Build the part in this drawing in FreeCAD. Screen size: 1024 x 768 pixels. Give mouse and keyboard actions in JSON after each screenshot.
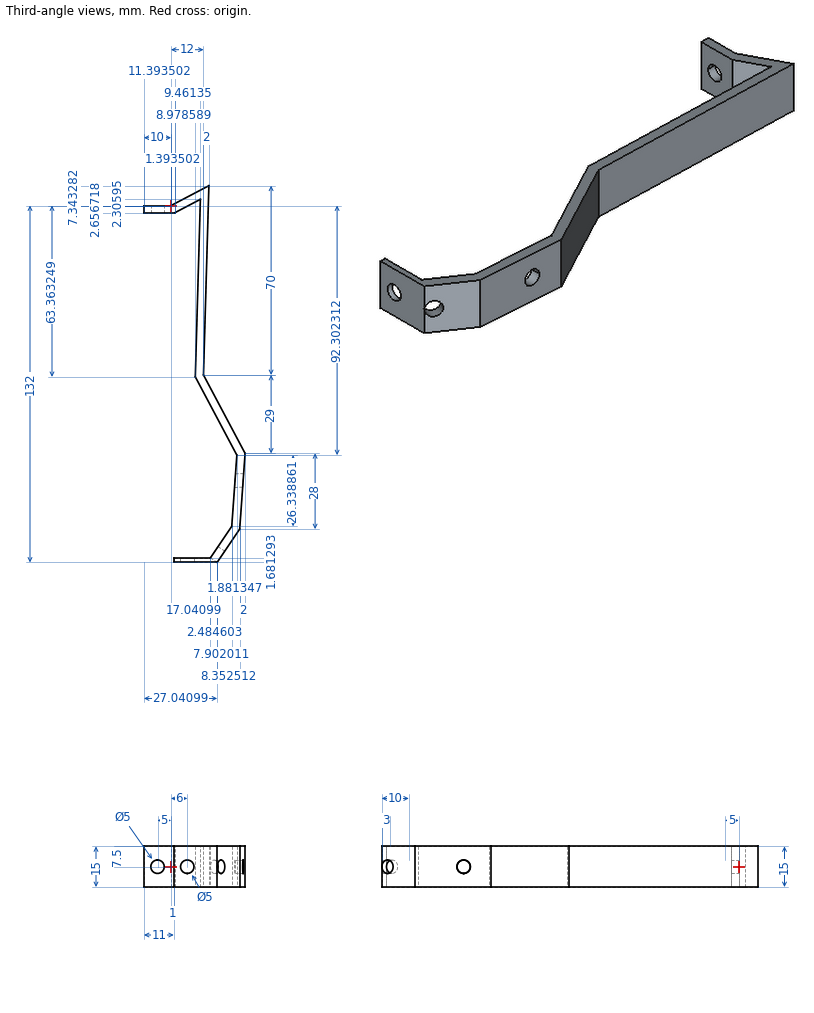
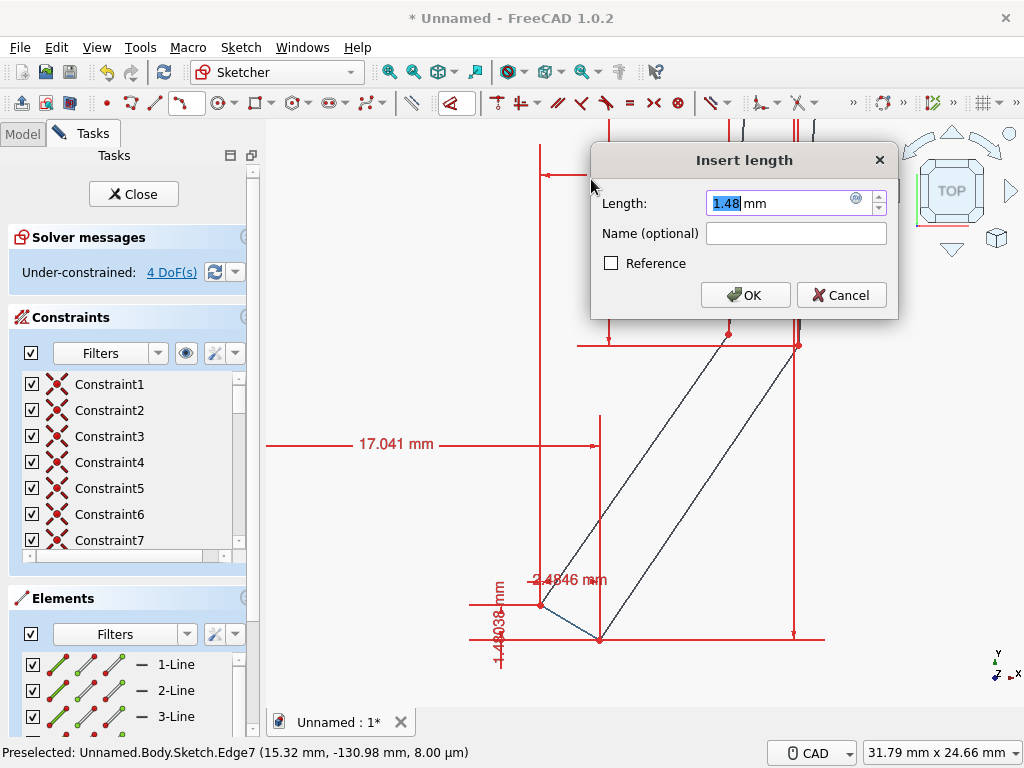
{"action": "type", "text": "1.681293"}
{"action": "key", "text": "Return"}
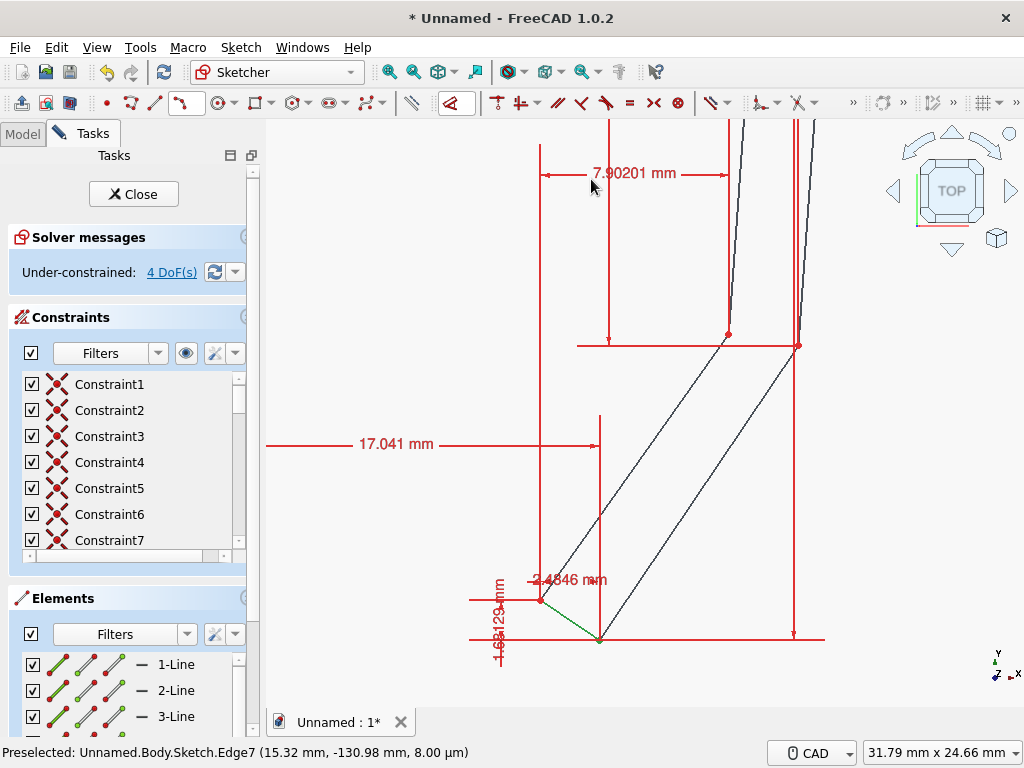
{"action": "scroll", "coordinate": [584, 592], "scroll_direction": "down", "scroll_amount": 11}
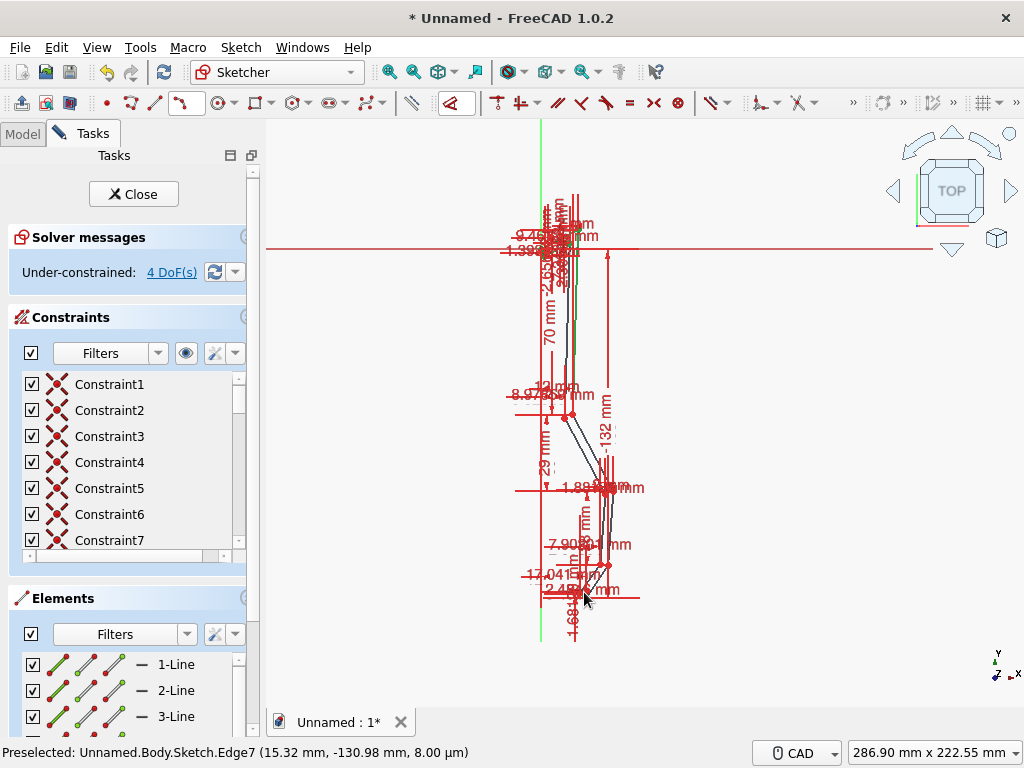
{"action": "scroll", "coordinate": [593, 588], "scroll_direction": "up", "scroll_amount": 3}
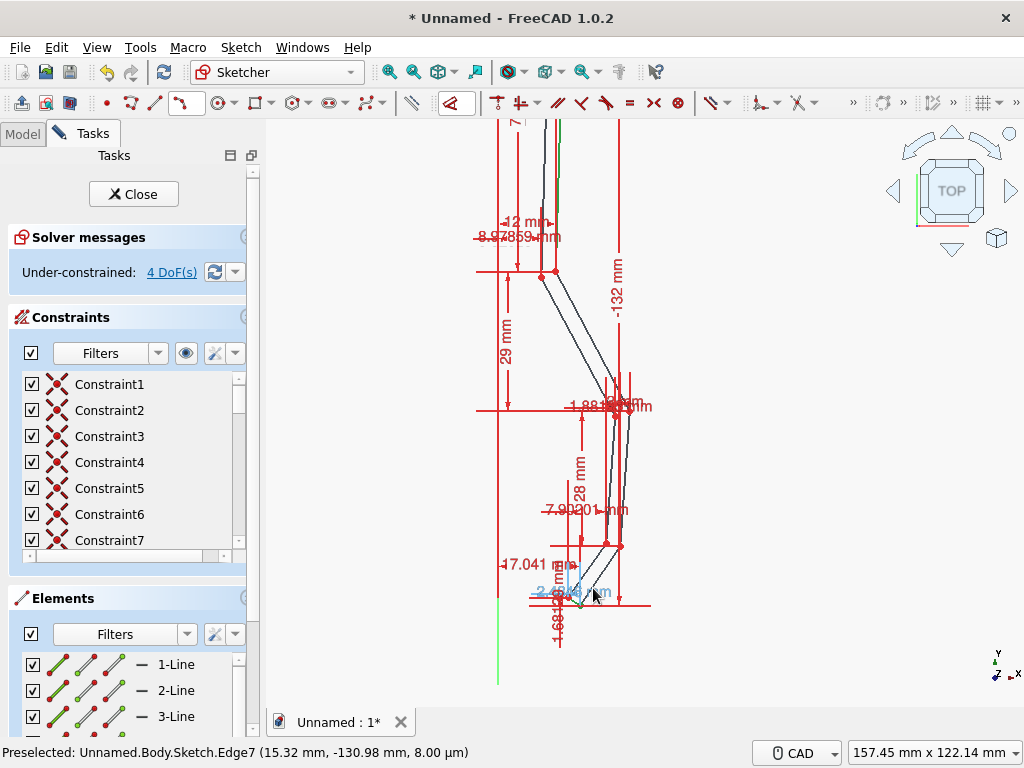
{"action": "left_click", "coordinate": [608, 564]}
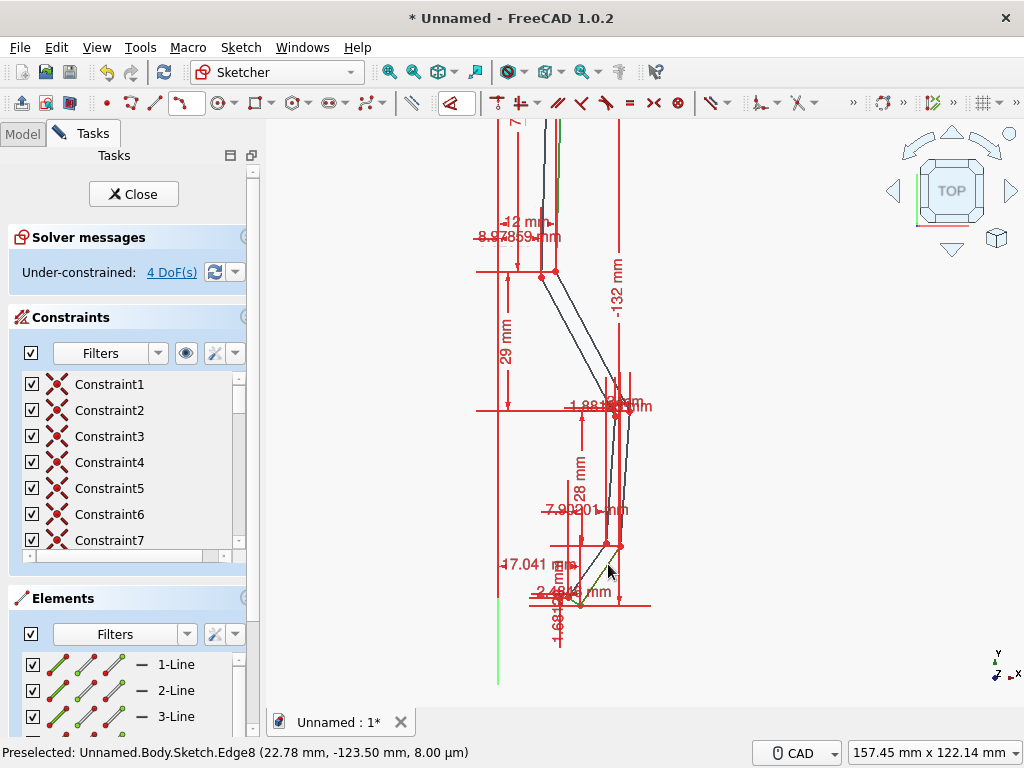
{"action": "left_click", "coordinate": [470, 104]}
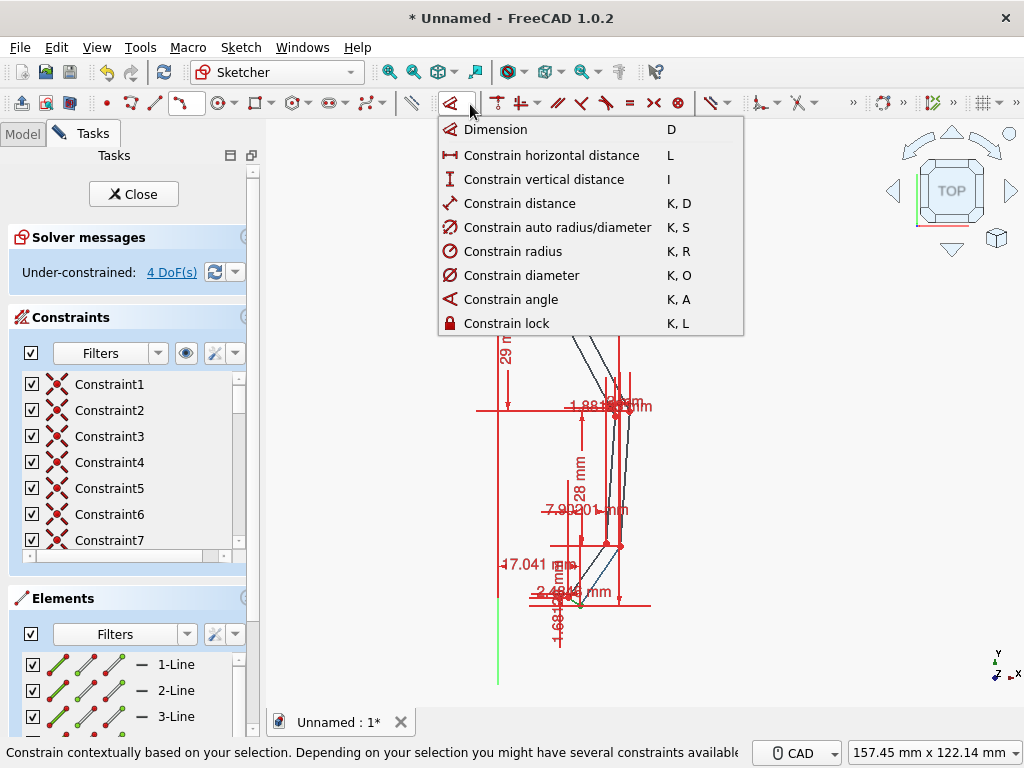
{"action": "left_click", "coordinate": [591, 155]}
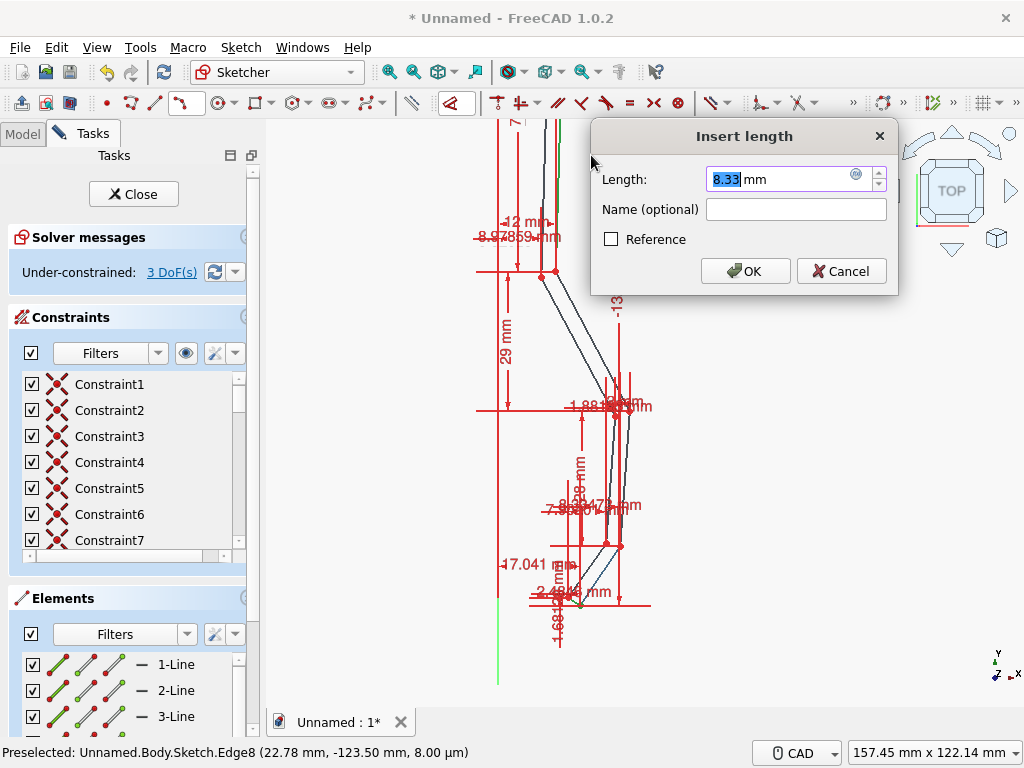
{"action": "type", "text": "8.352512"}
{"action": "key", "text": "Return"}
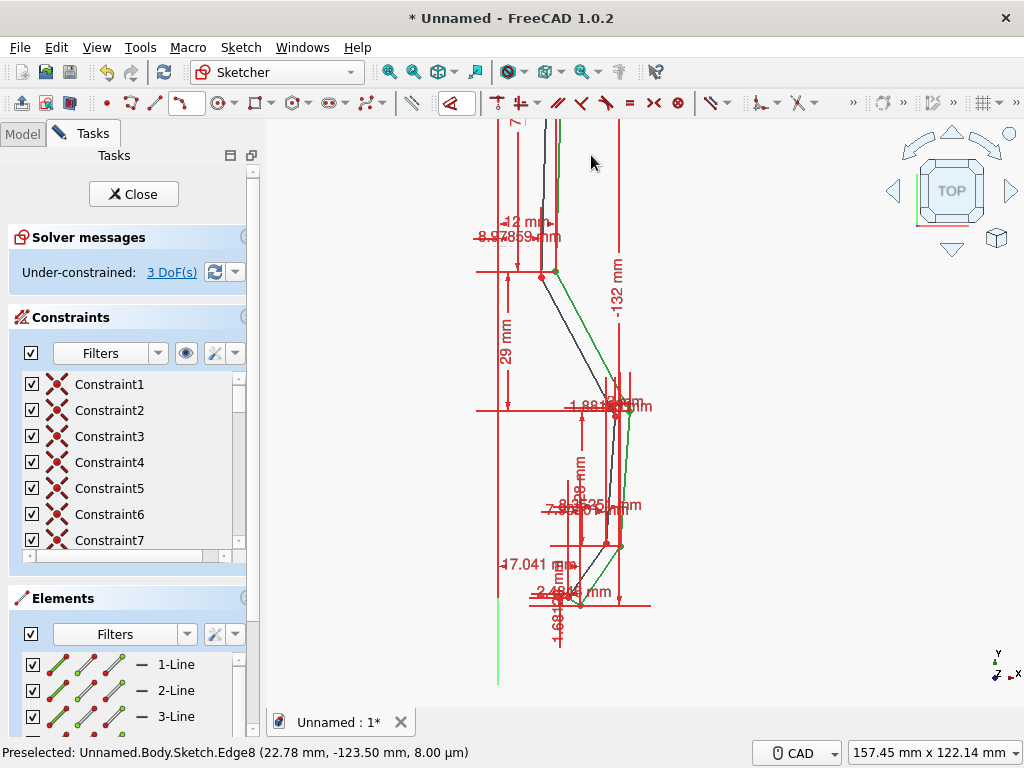
{"action": "left_click", "coordinate": [541, 278]}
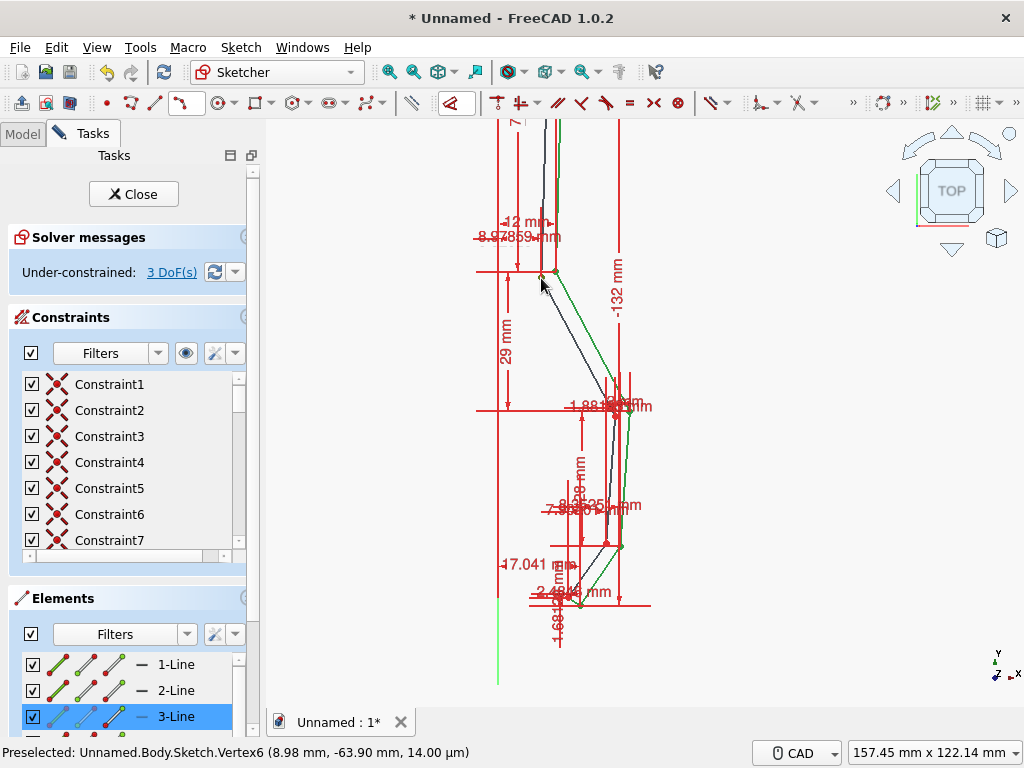
{"action": "left_click", "coordinate": [470, 104]}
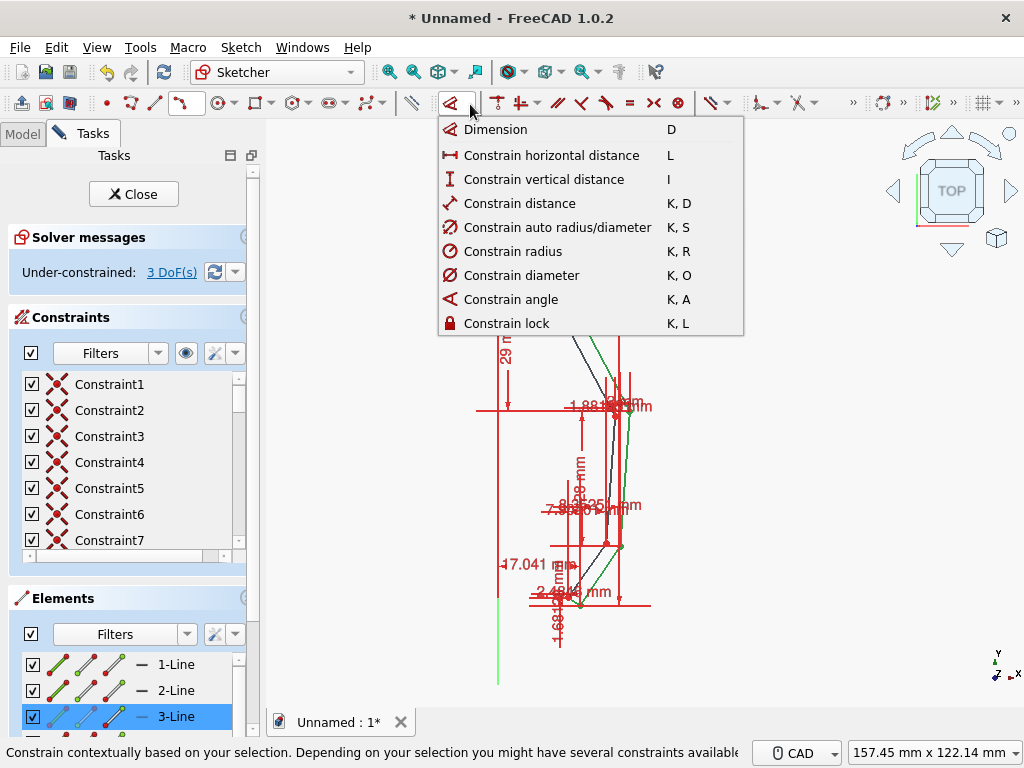
{"action": "left_click", "coordinate": [591, 179]}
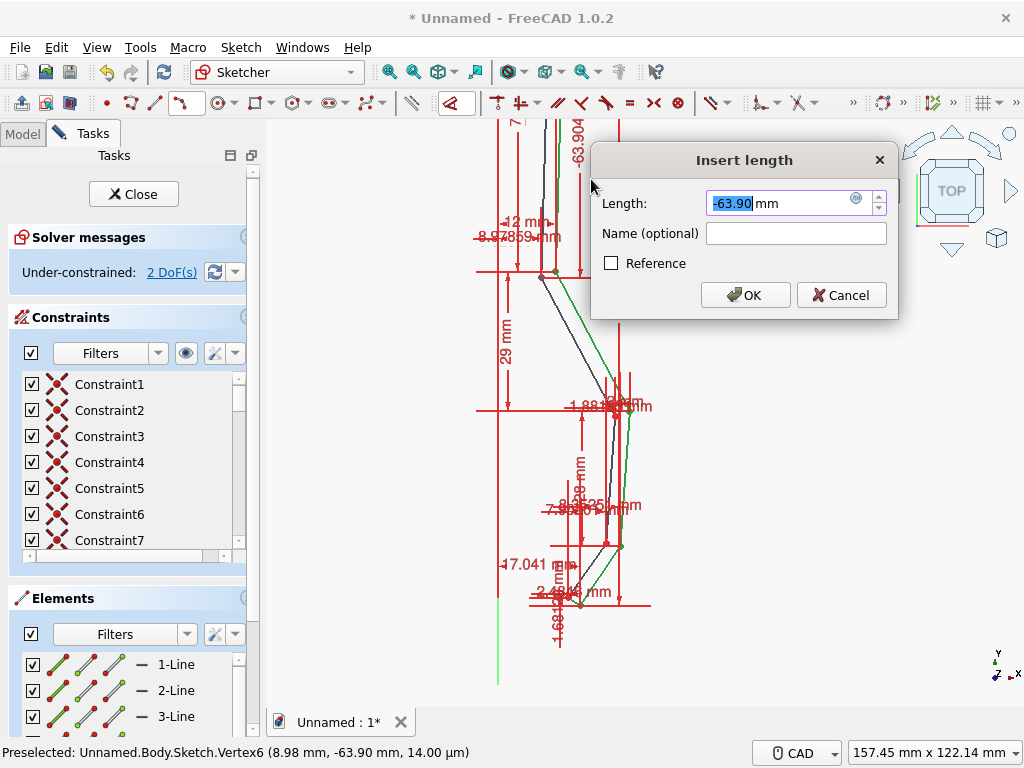
{"action": "type", "text": "-63.363249"}
{"action": "key", "text": "Return"}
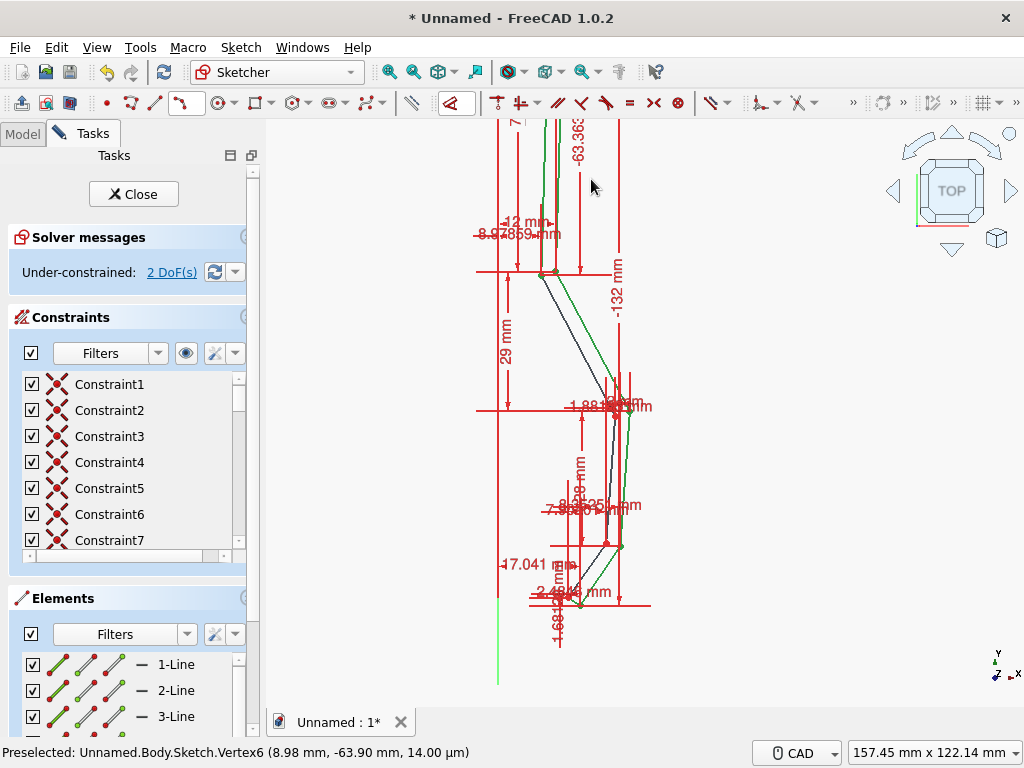
{"action": "left_click", "coordinate": [615, 416]}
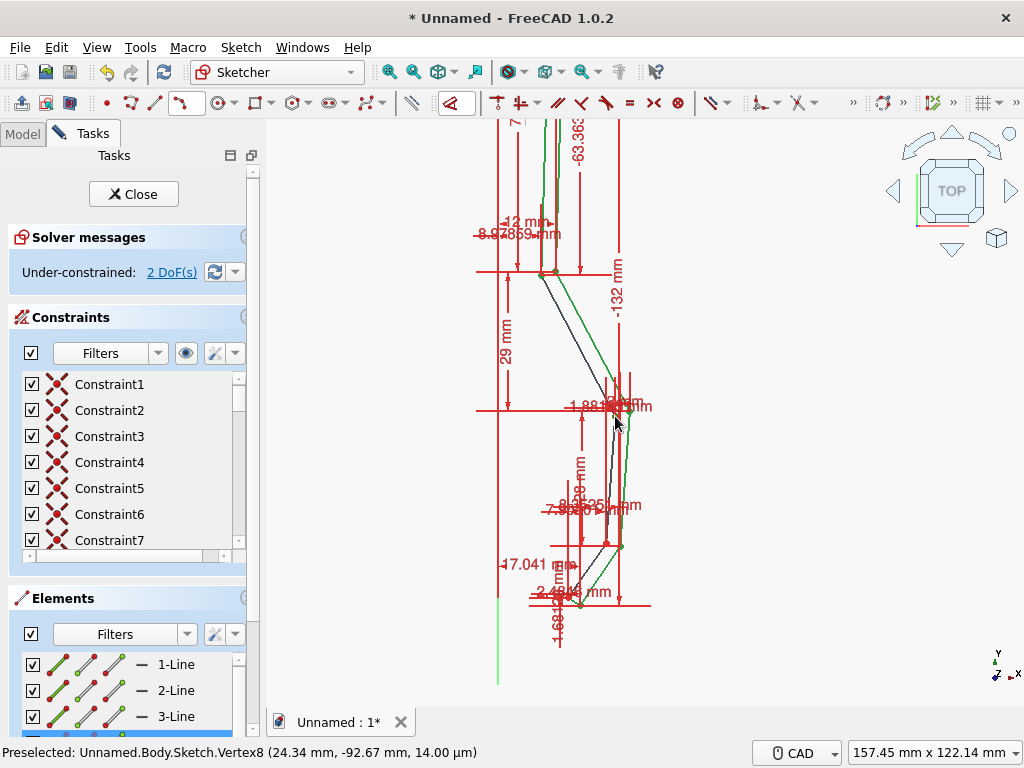
{"action": "key", "text": "i"}